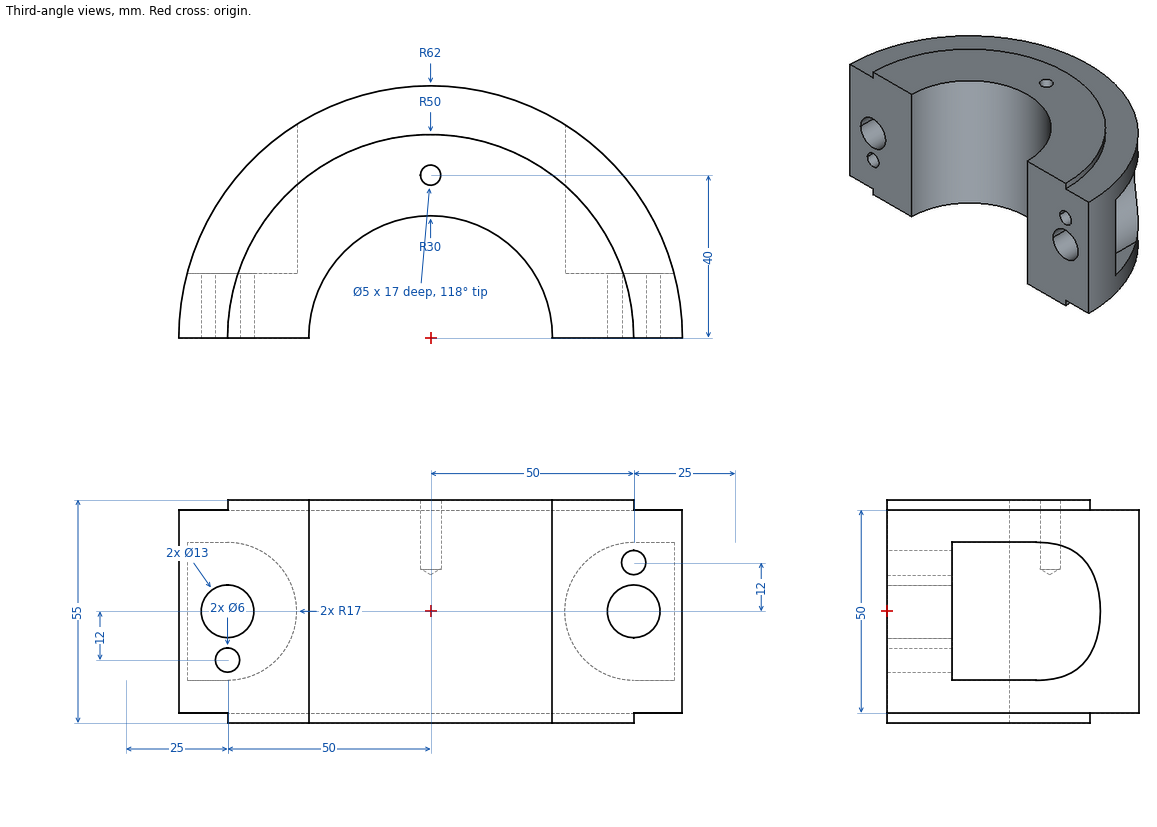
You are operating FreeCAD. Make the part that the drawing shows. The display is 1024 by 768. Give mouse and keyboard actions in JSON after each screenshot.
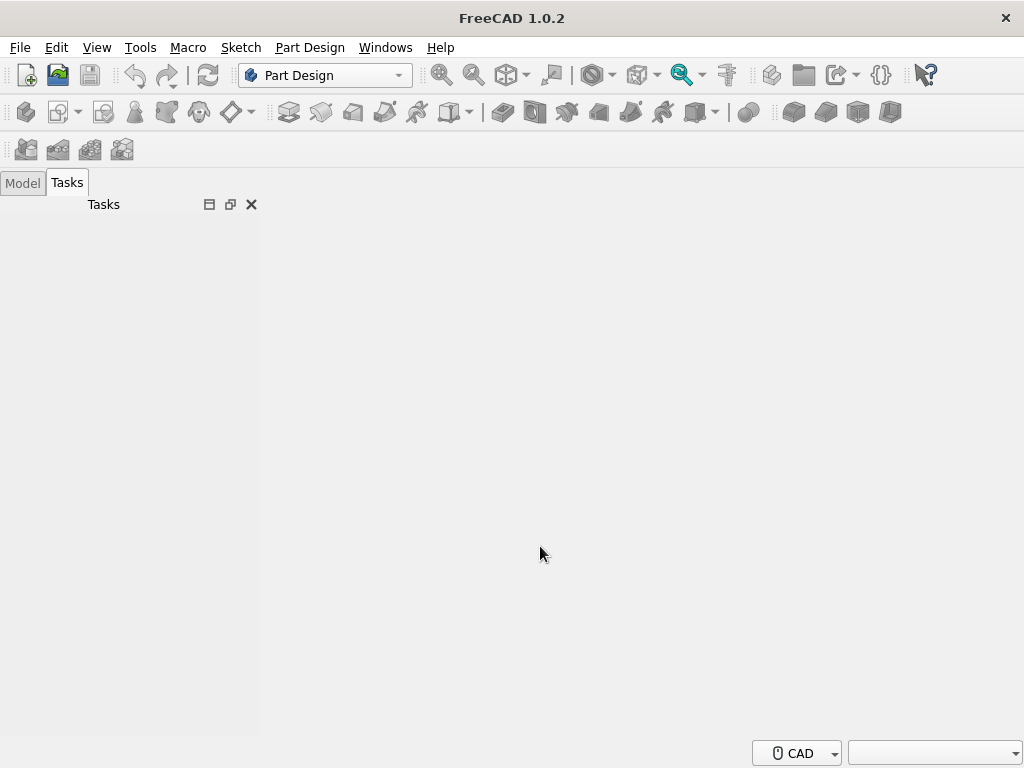
{"action": "left_click", "coordinate": [26, 76]}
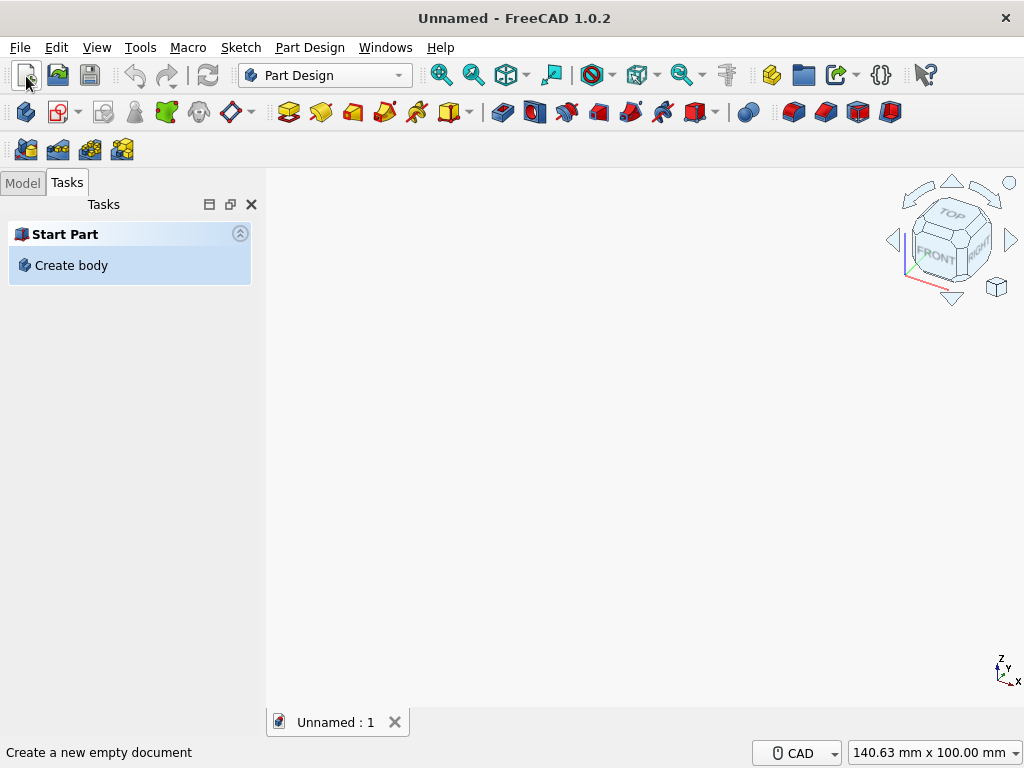
{"action": "left_click", "coordinate": [58, 112]}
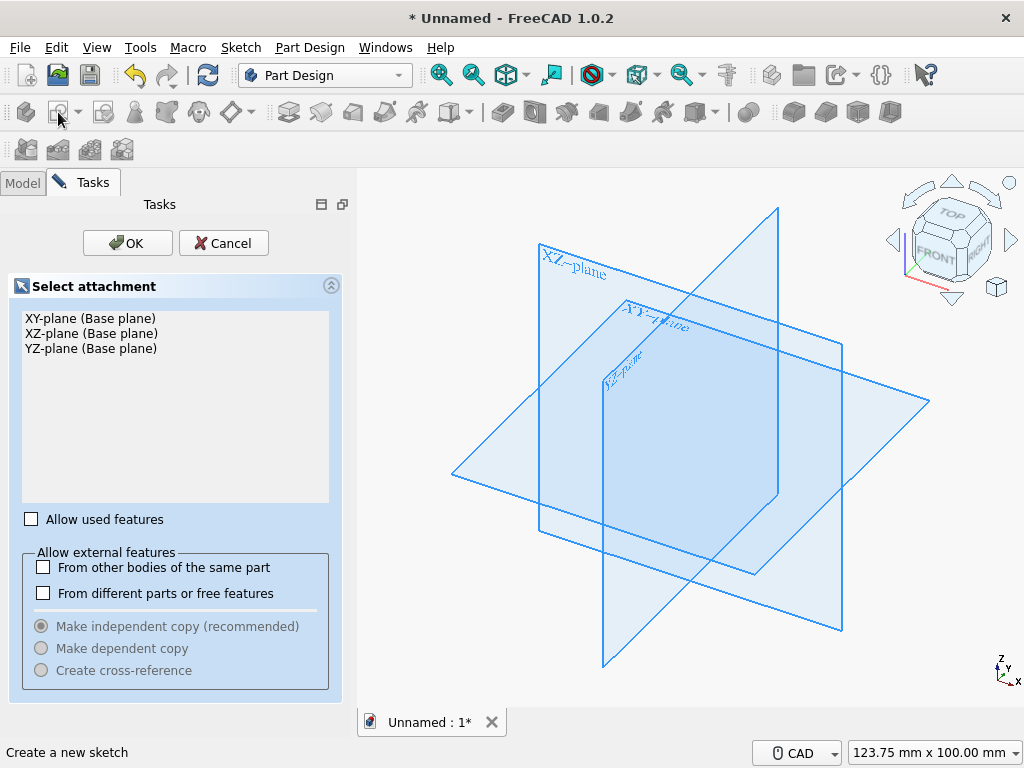
{"action": "left_click", "coordinate": [82, 318]}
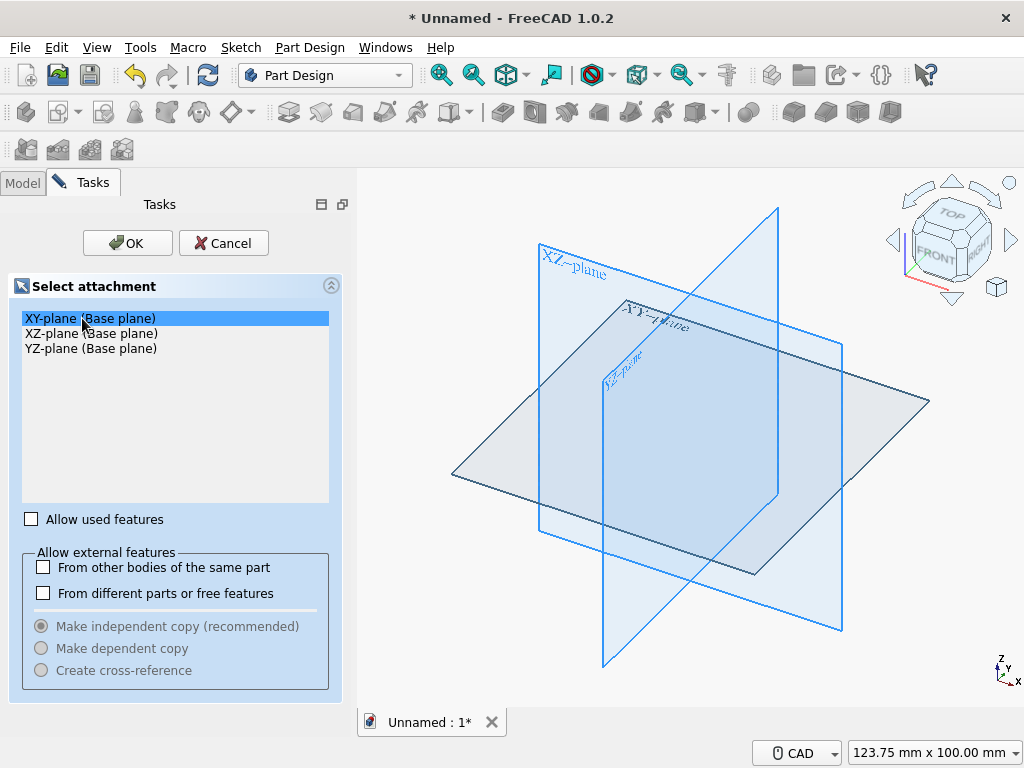
{"action": "left_click", "coordinate": [128, 243]}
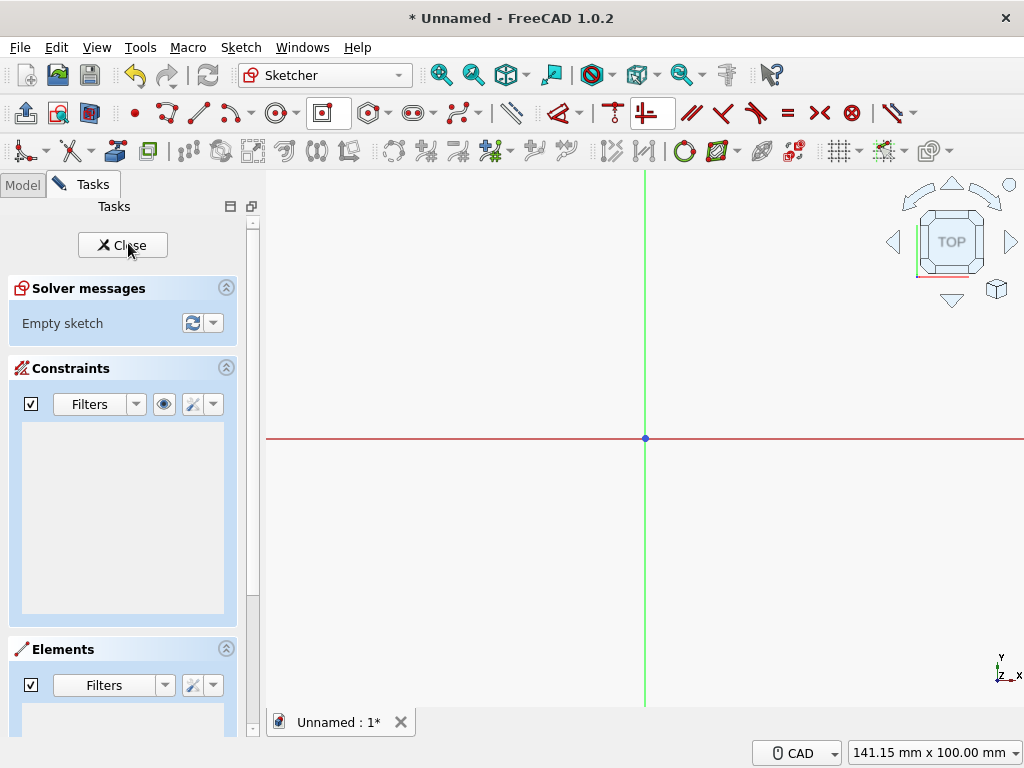
{"action": "scroll", "coordinate": [493, 641], "scroll_direction": "down", "scroll_amount": 3}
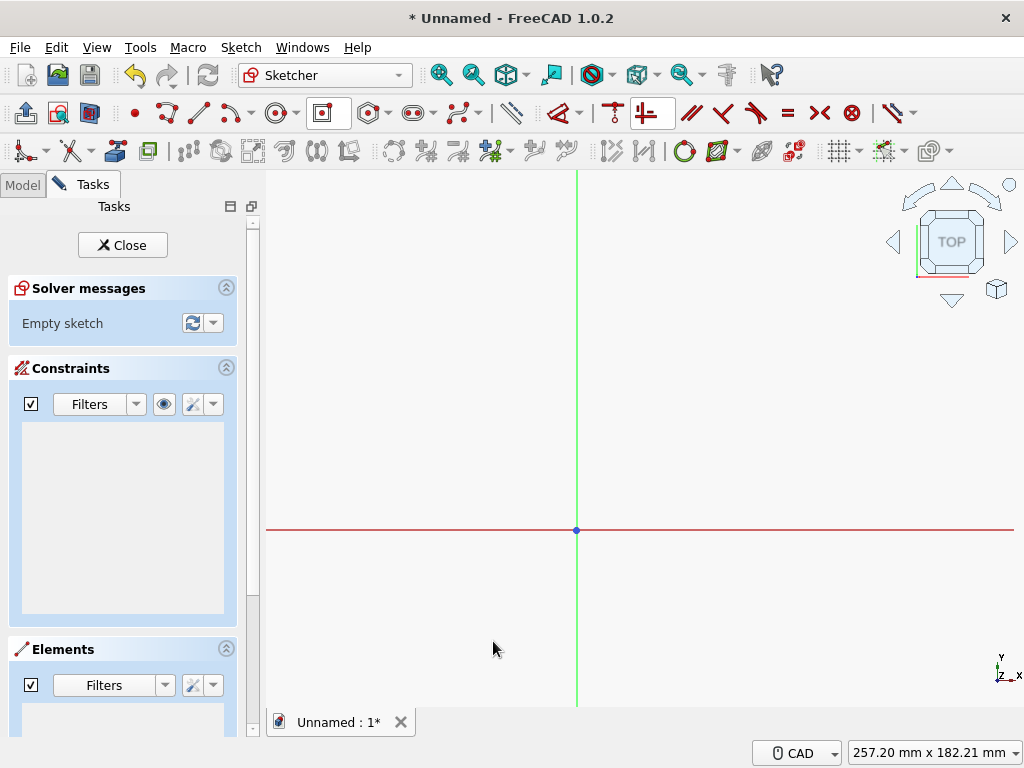
{"action": "left_click", "coordinate": [200, 114]}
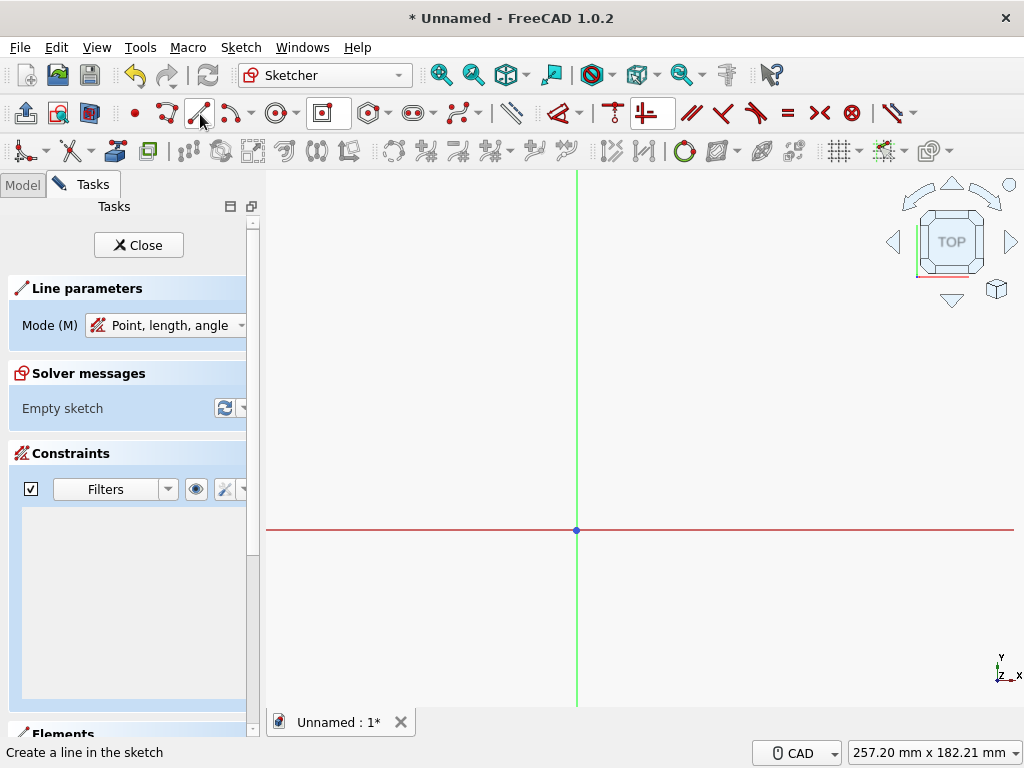
{"action": "left_click", "coordinate": [394, 530]}
{"action": "left_click", "coordinate": [488, 521]}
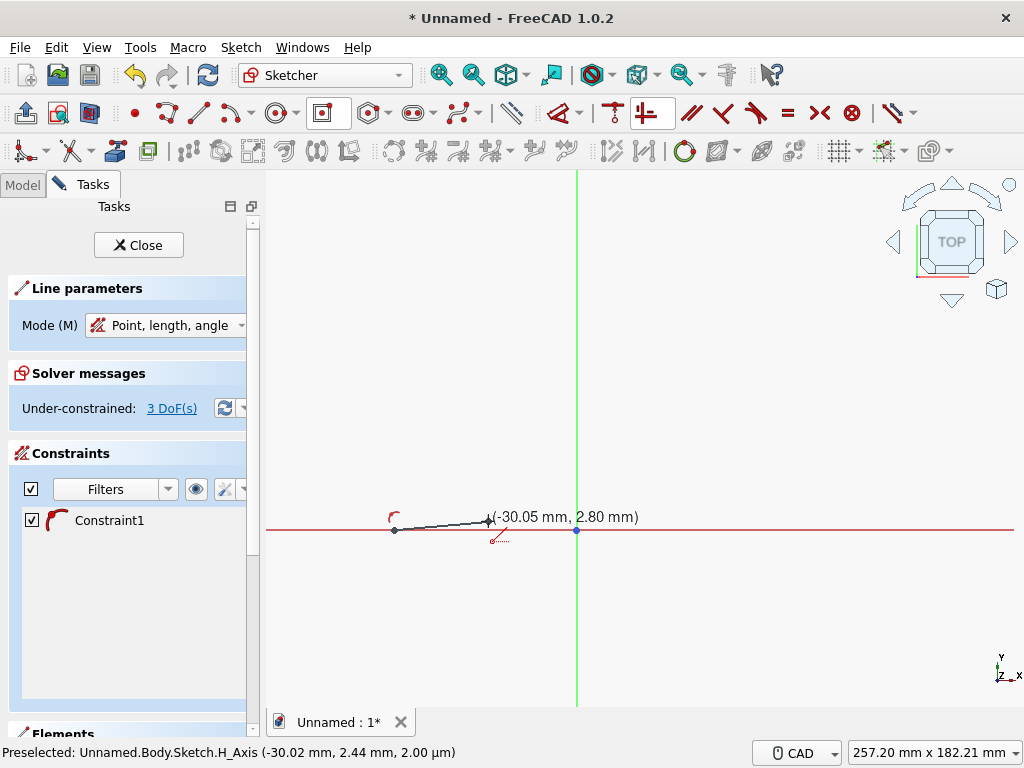
{"action": "left_click", "coordinate": [665, 530]}
{"action": "left_click", "coordinate": [759, 521]}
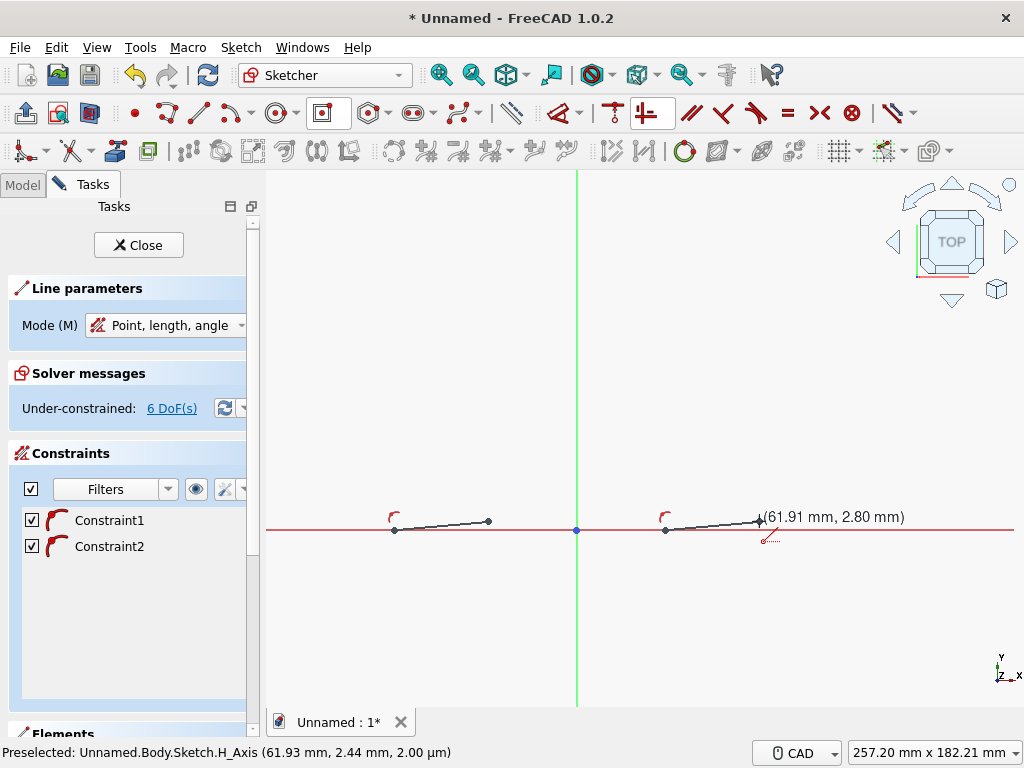
{"action": "left_click", "coordinate": [254, 114]}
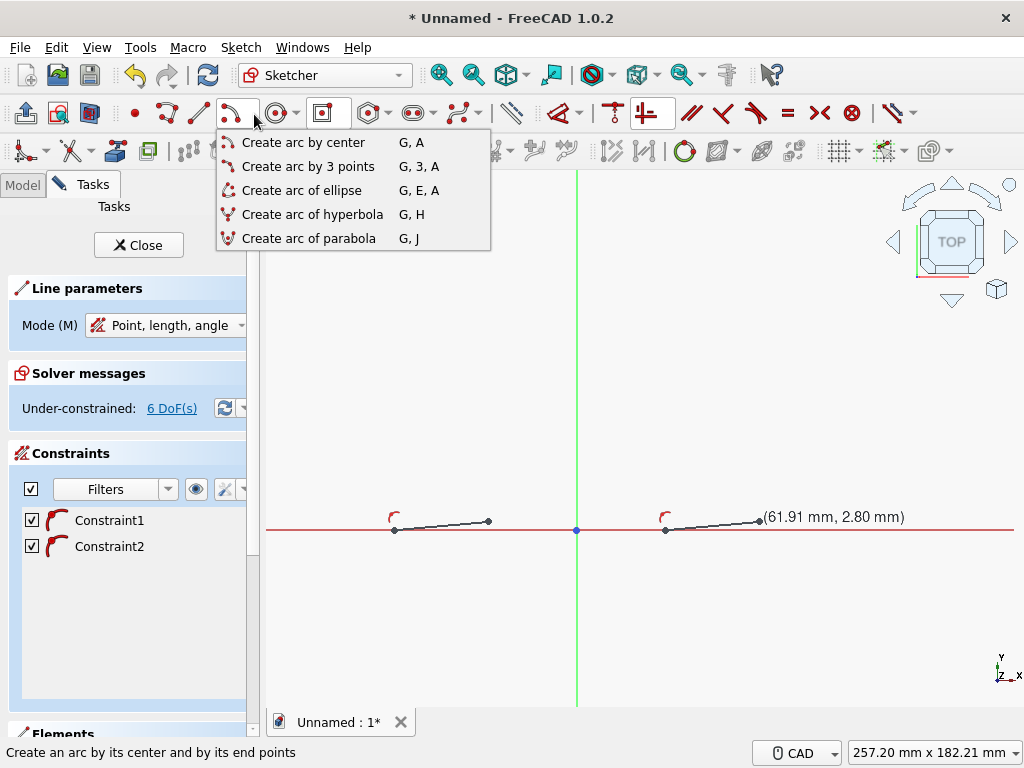
{"action": "left_click", "coordinate": [354, 166]}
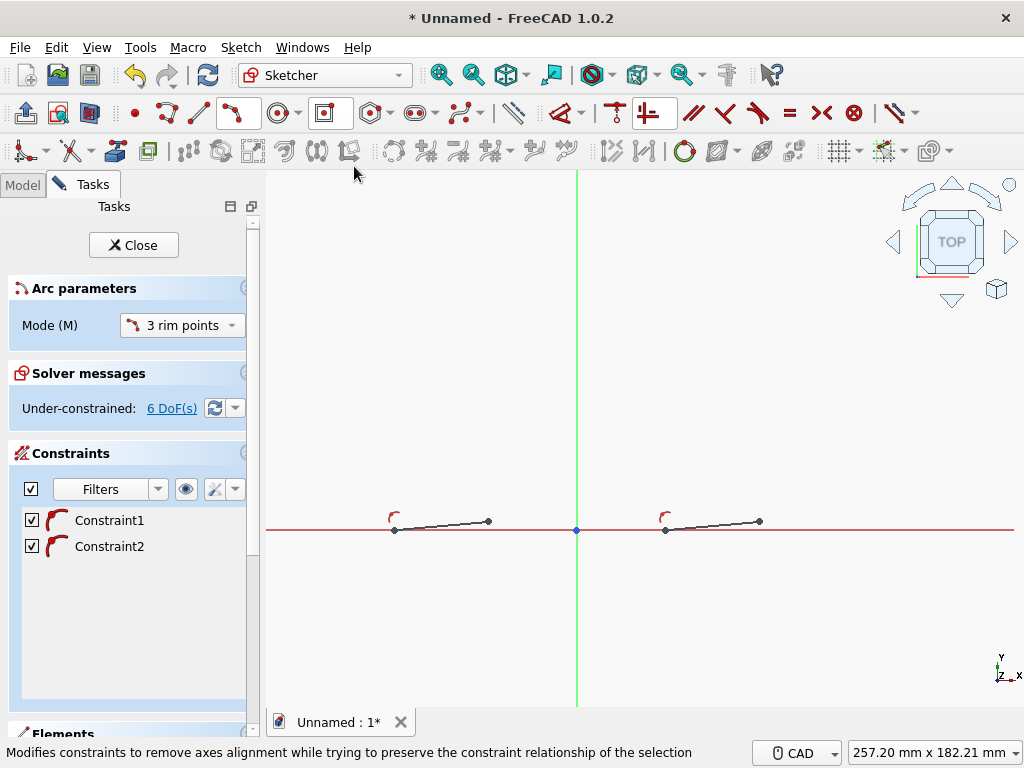
{"action": "left_click", "coordinate": [488, 522]}
{"action": "left_click", "coordinate": [665, 530]}
{"action": "left_click", "coordinate": [604, 446]}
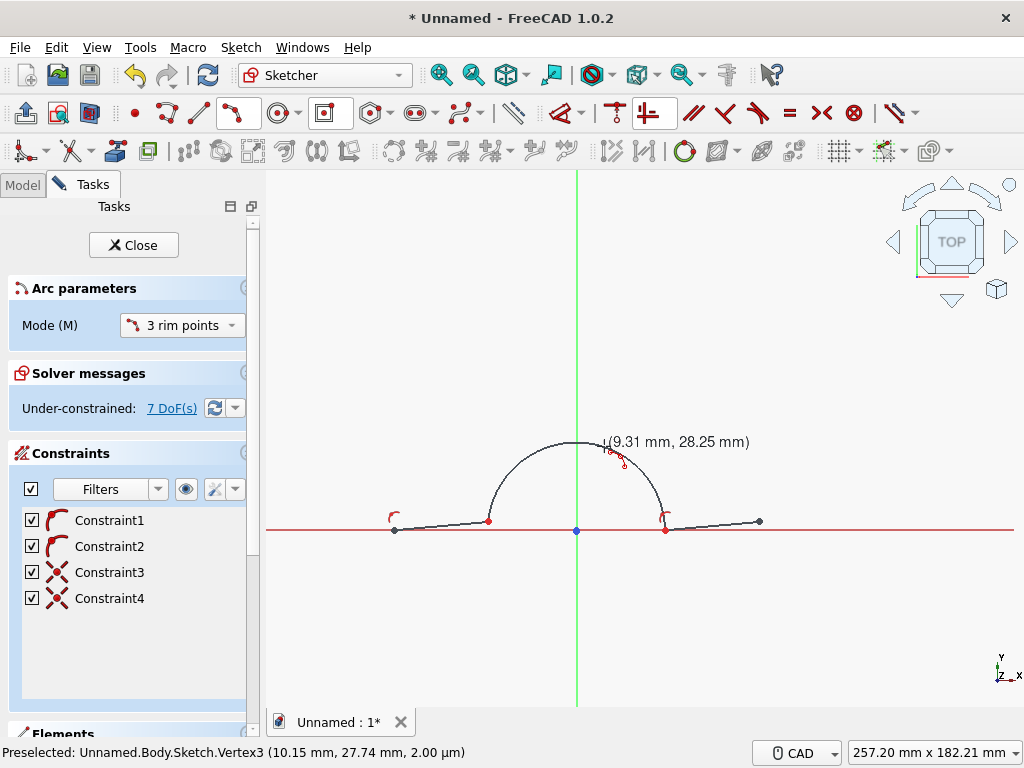
{"action": "left_click", "coordinate": [759, 522]}
{"action": "left_click", "coordinate": [394, 530]}
{"action": "left_click", "coordinate": [633, 356]}
{"action": "key", "text": "Escape"}